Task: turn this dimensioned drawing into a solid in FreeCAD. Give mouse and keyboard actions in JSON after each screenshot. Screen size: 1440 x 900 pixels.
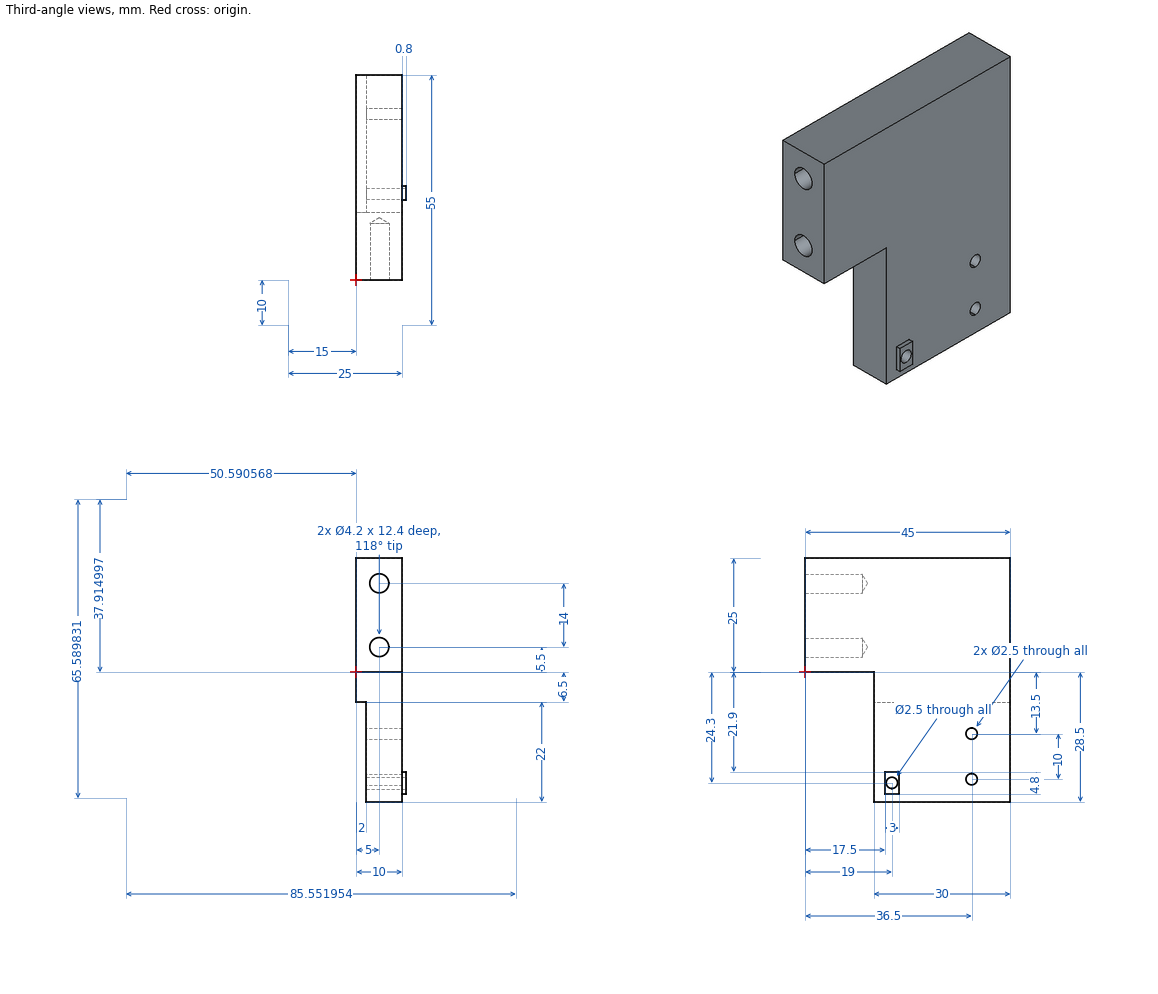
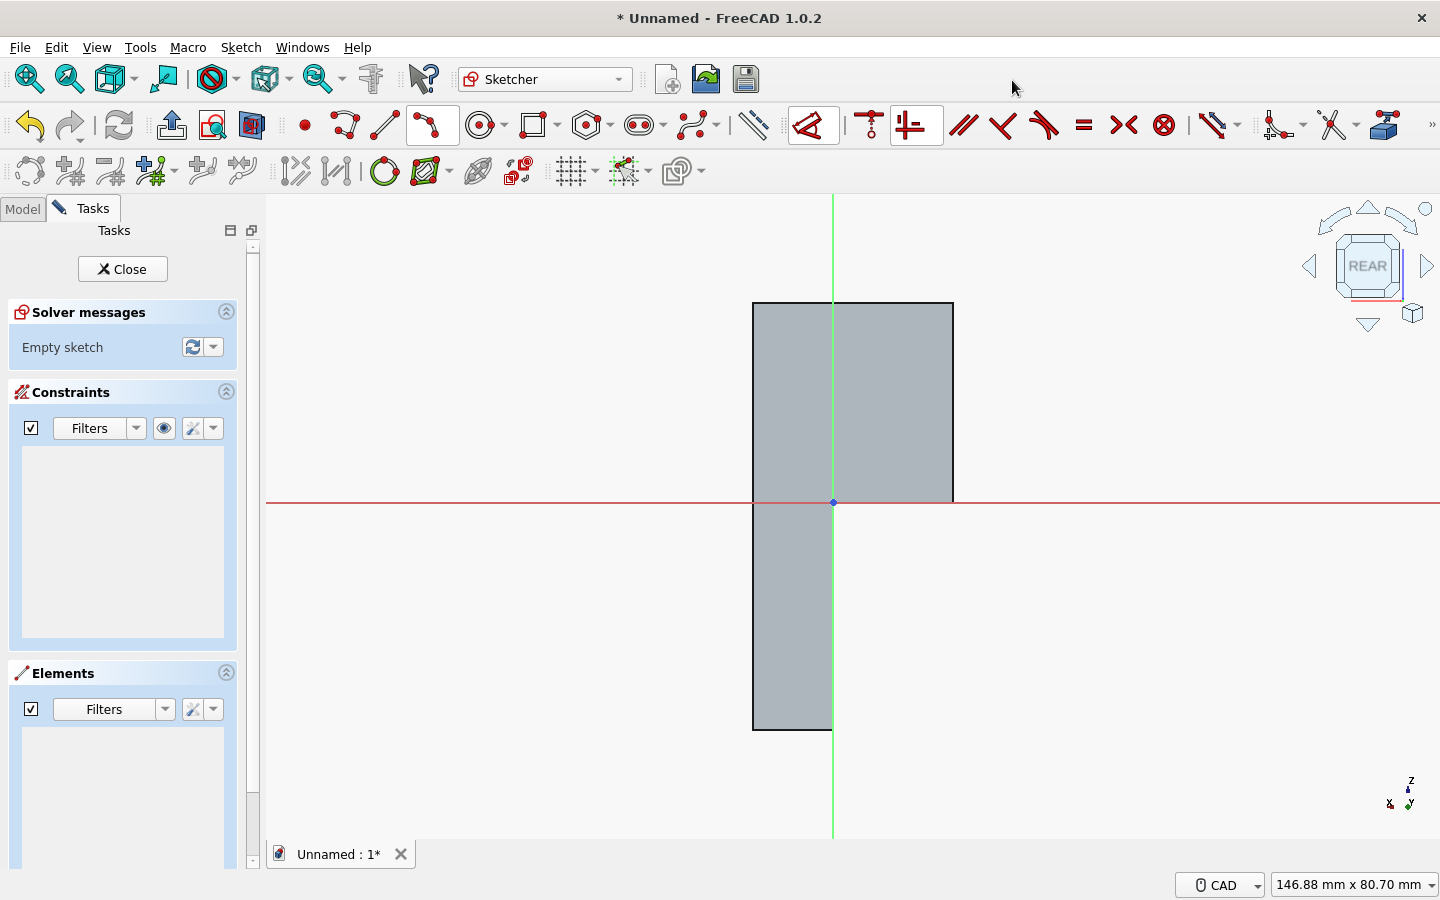
{"action": "scroll", "coordinate": [874, 738], "scroll_direction": "up", "scroll_amount": 3}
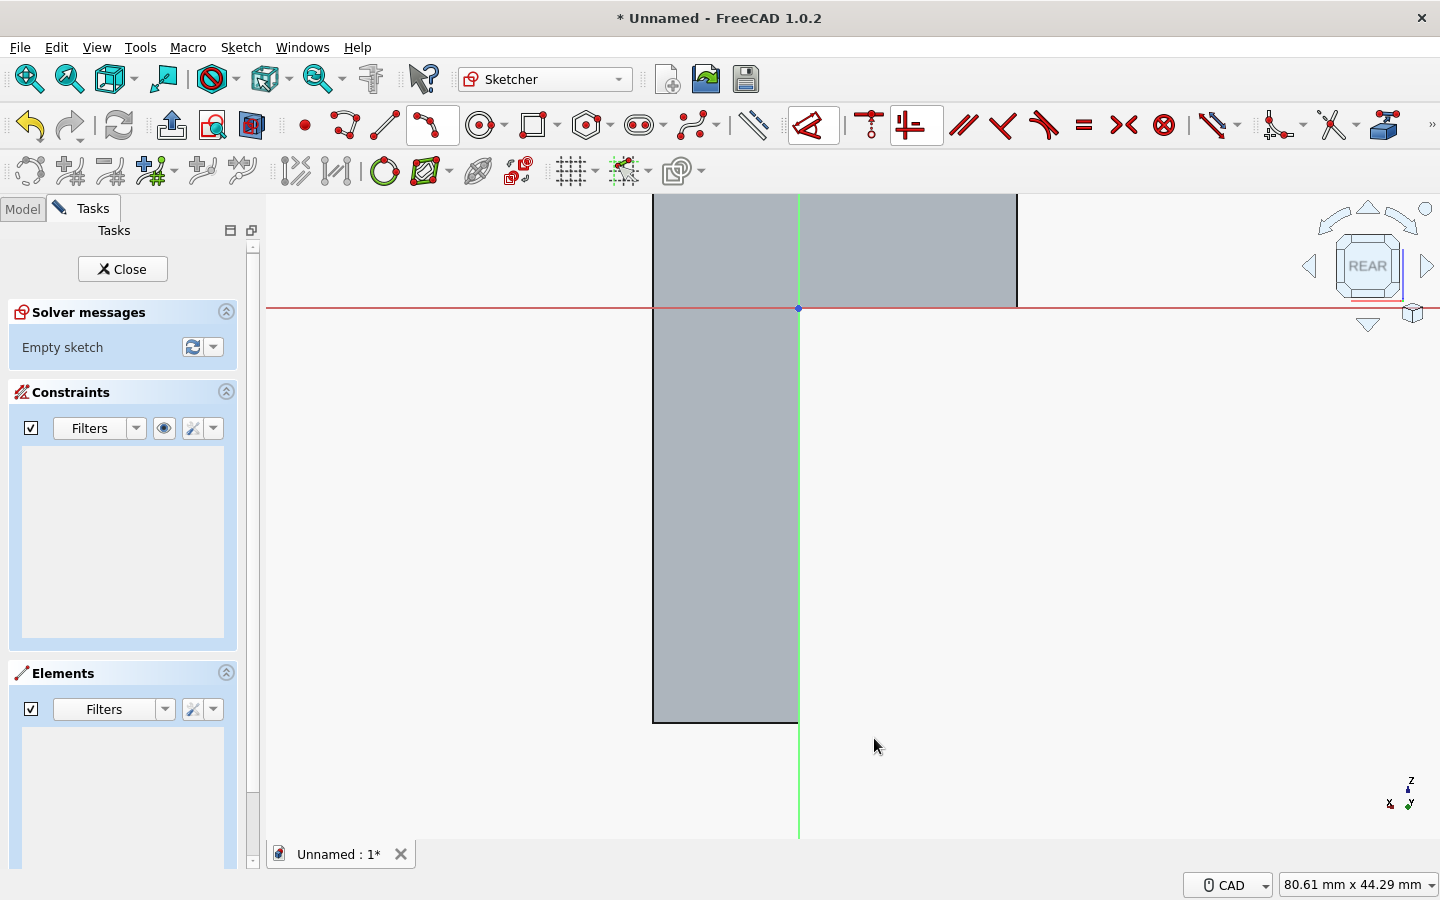
{"action": "key", "text": "g r"}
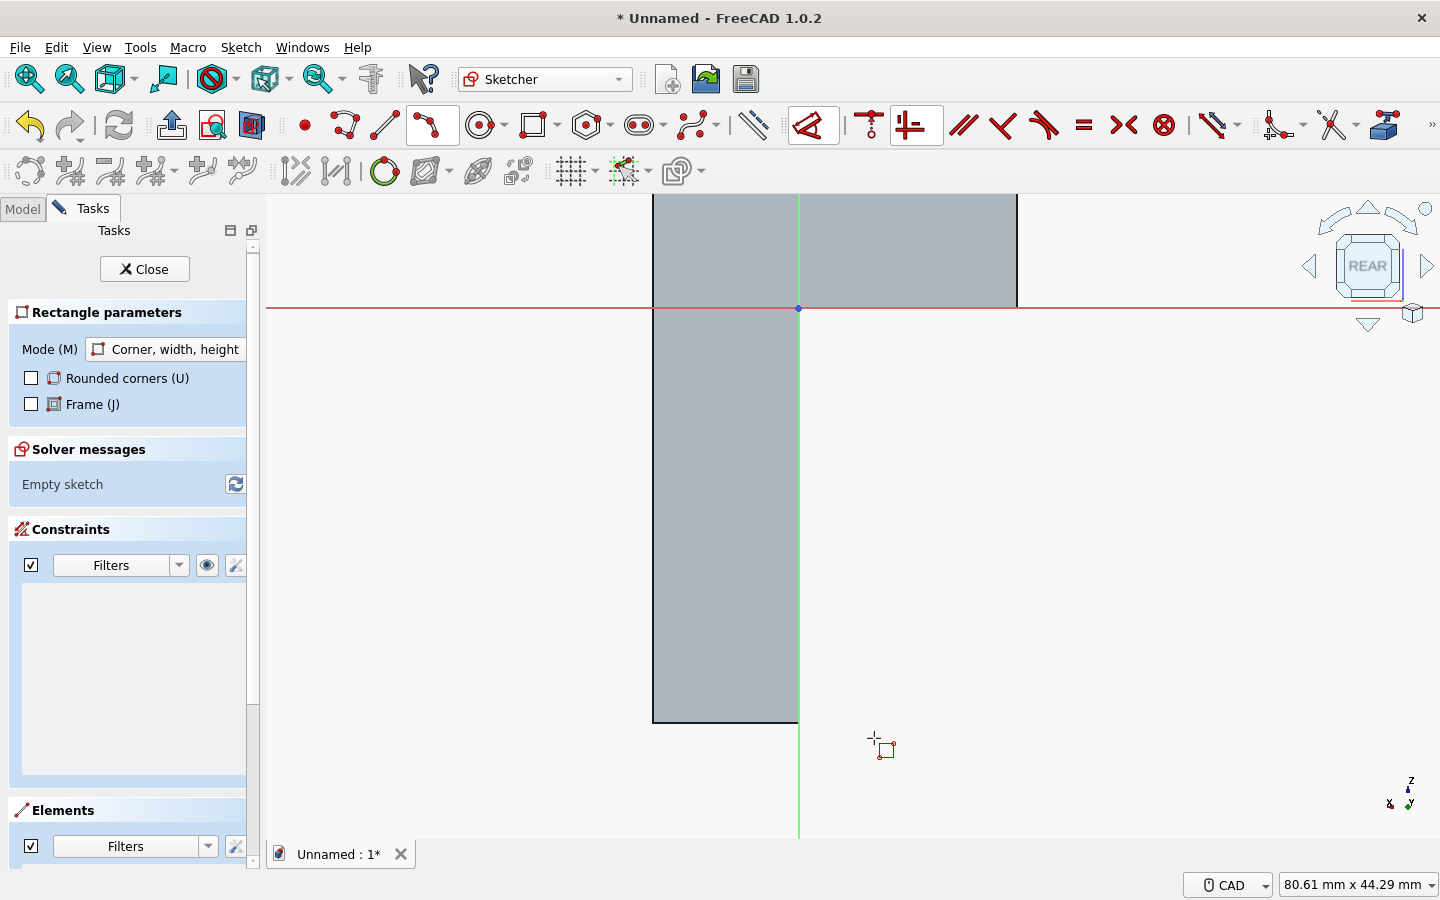
{"action": "left_click", "coordinate": [770, 403]}
{"action": "left_click", "coordinate": [799, 723]}
{"action": "key", "text": "Escape"}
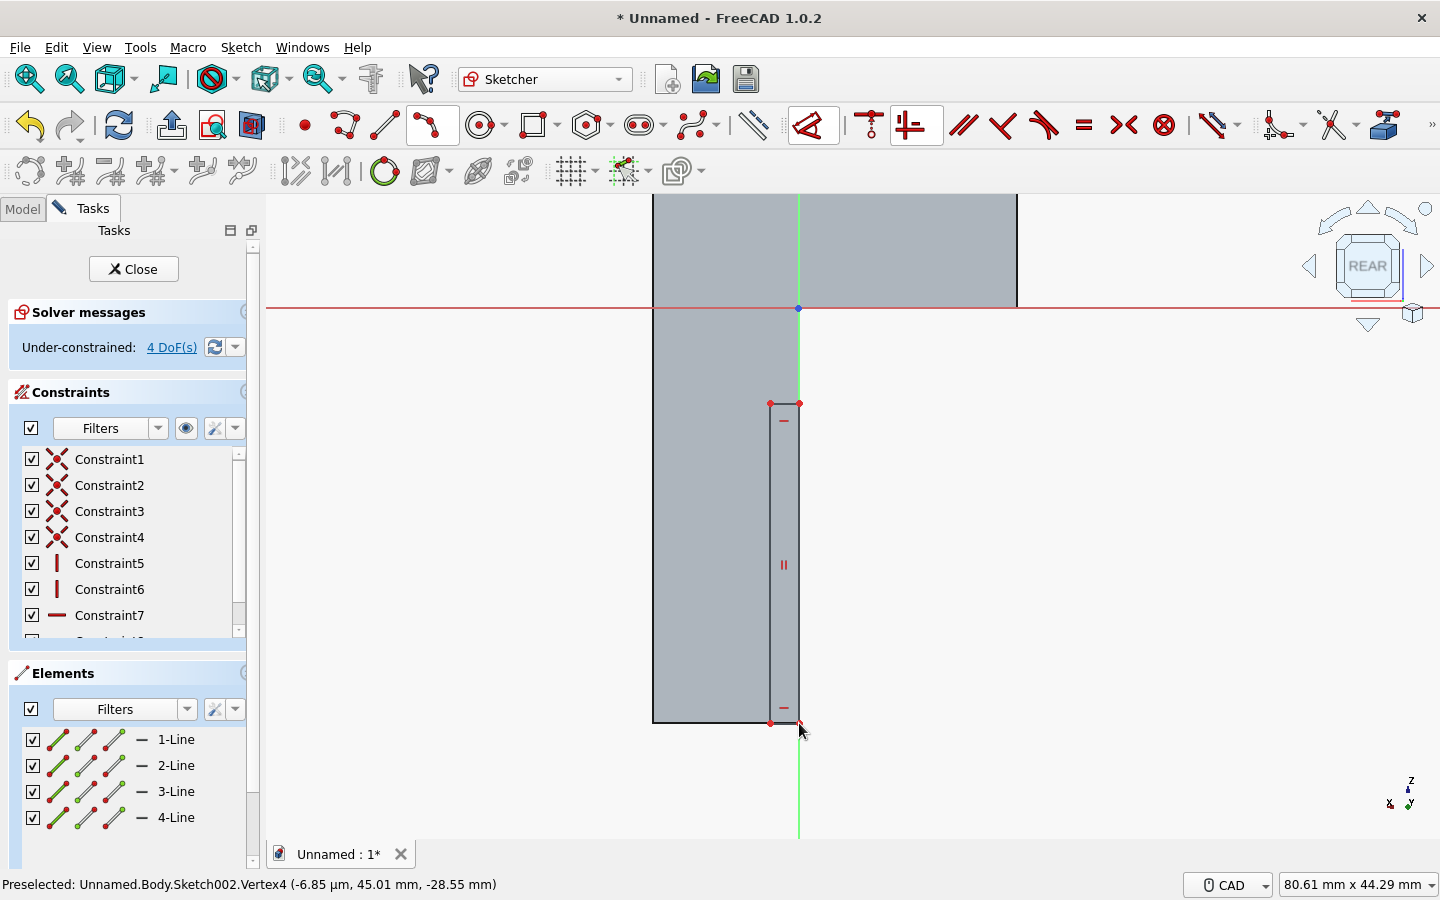
{"action": "left_click", "coordinate": [799, 724]}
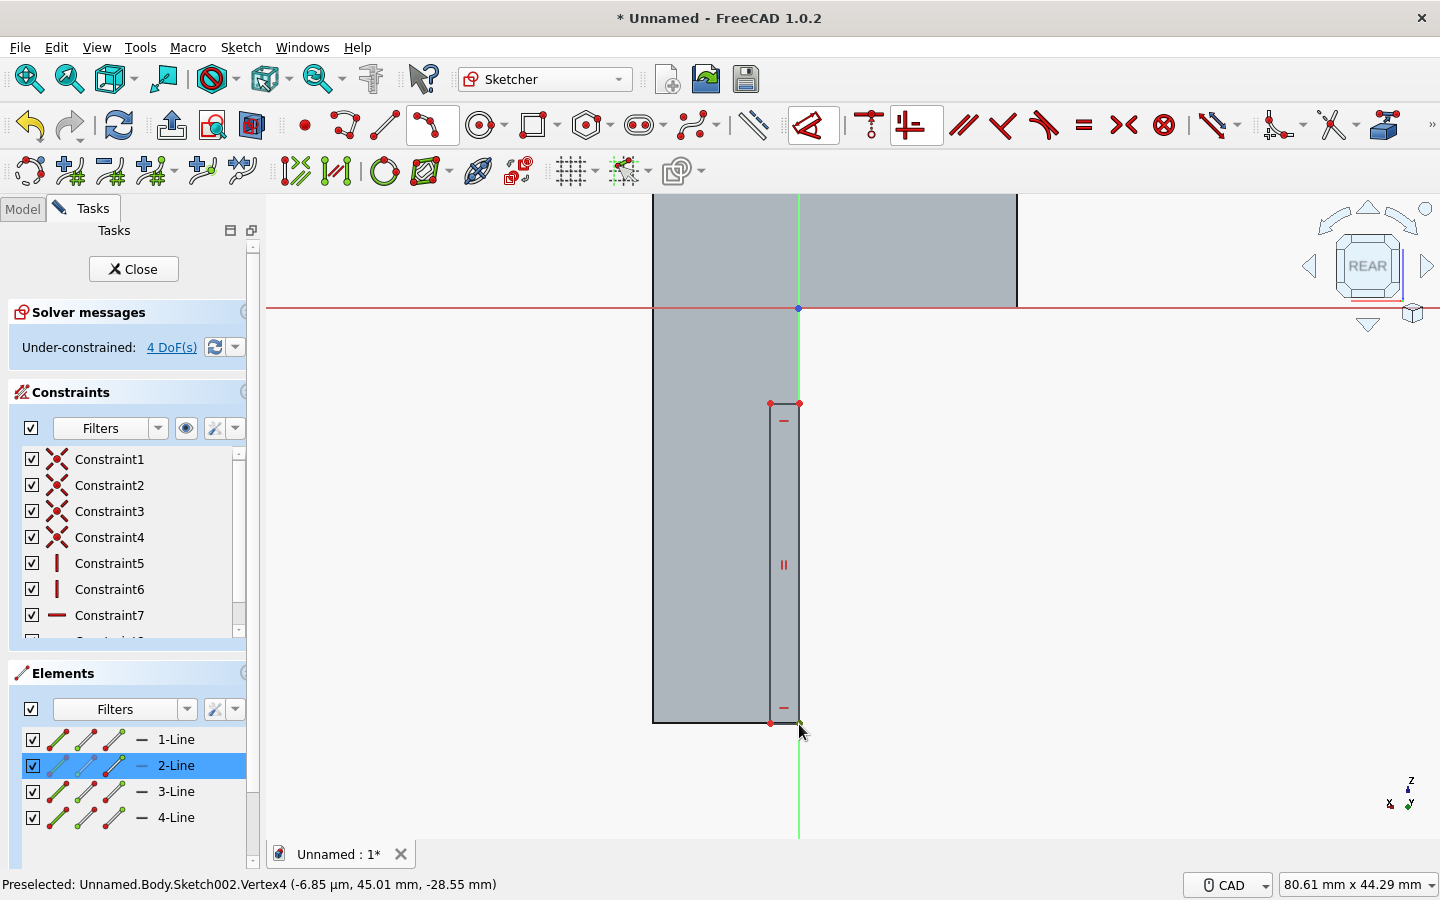
{"action": "left_click", "coordinate": [799, 769]}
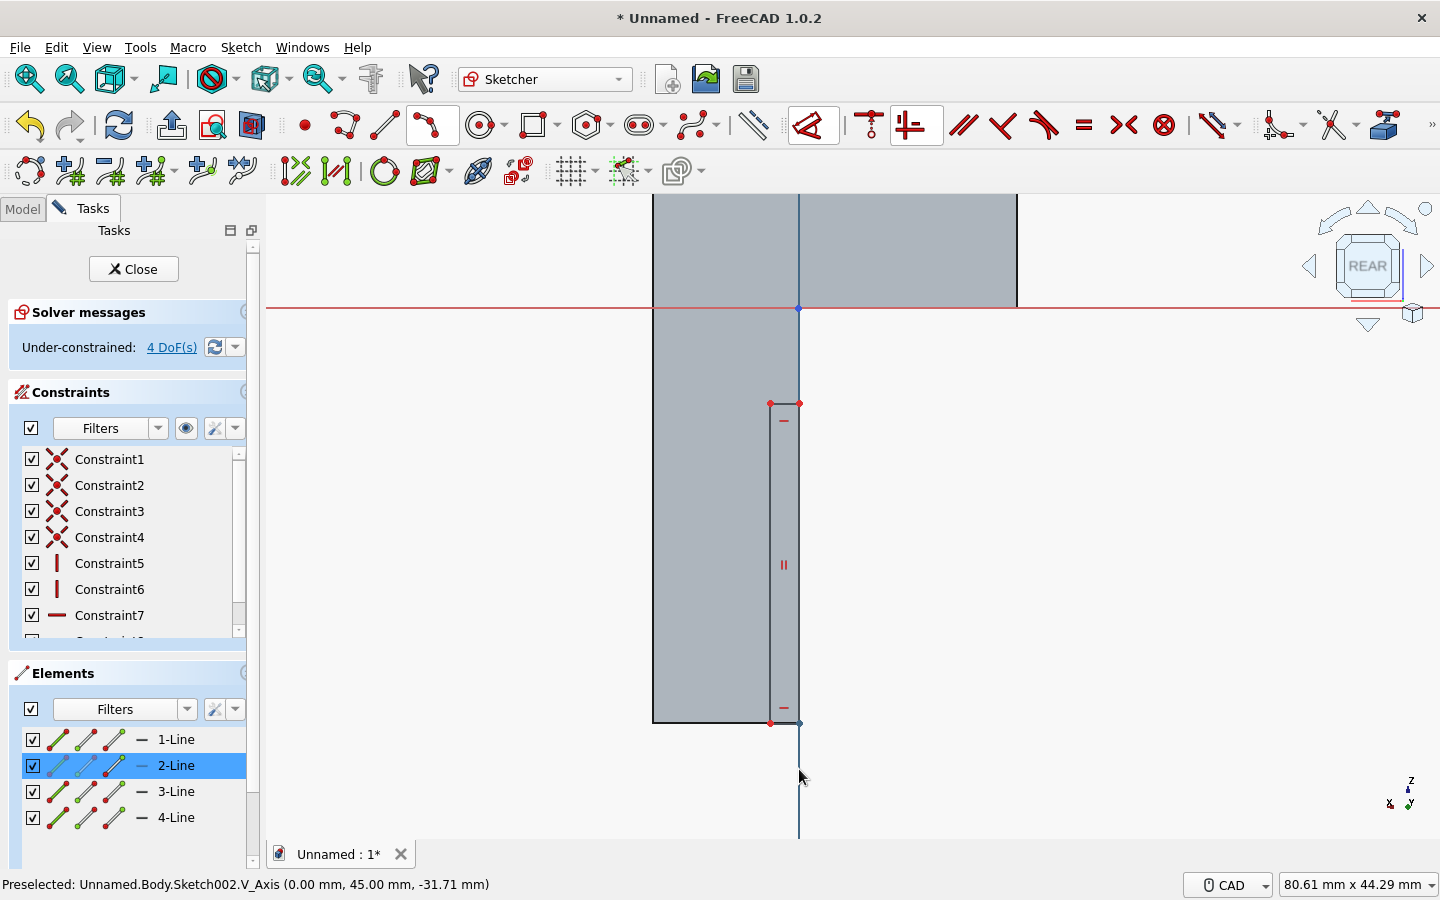
{"action": "left_click", "coordinate": [870, 126]}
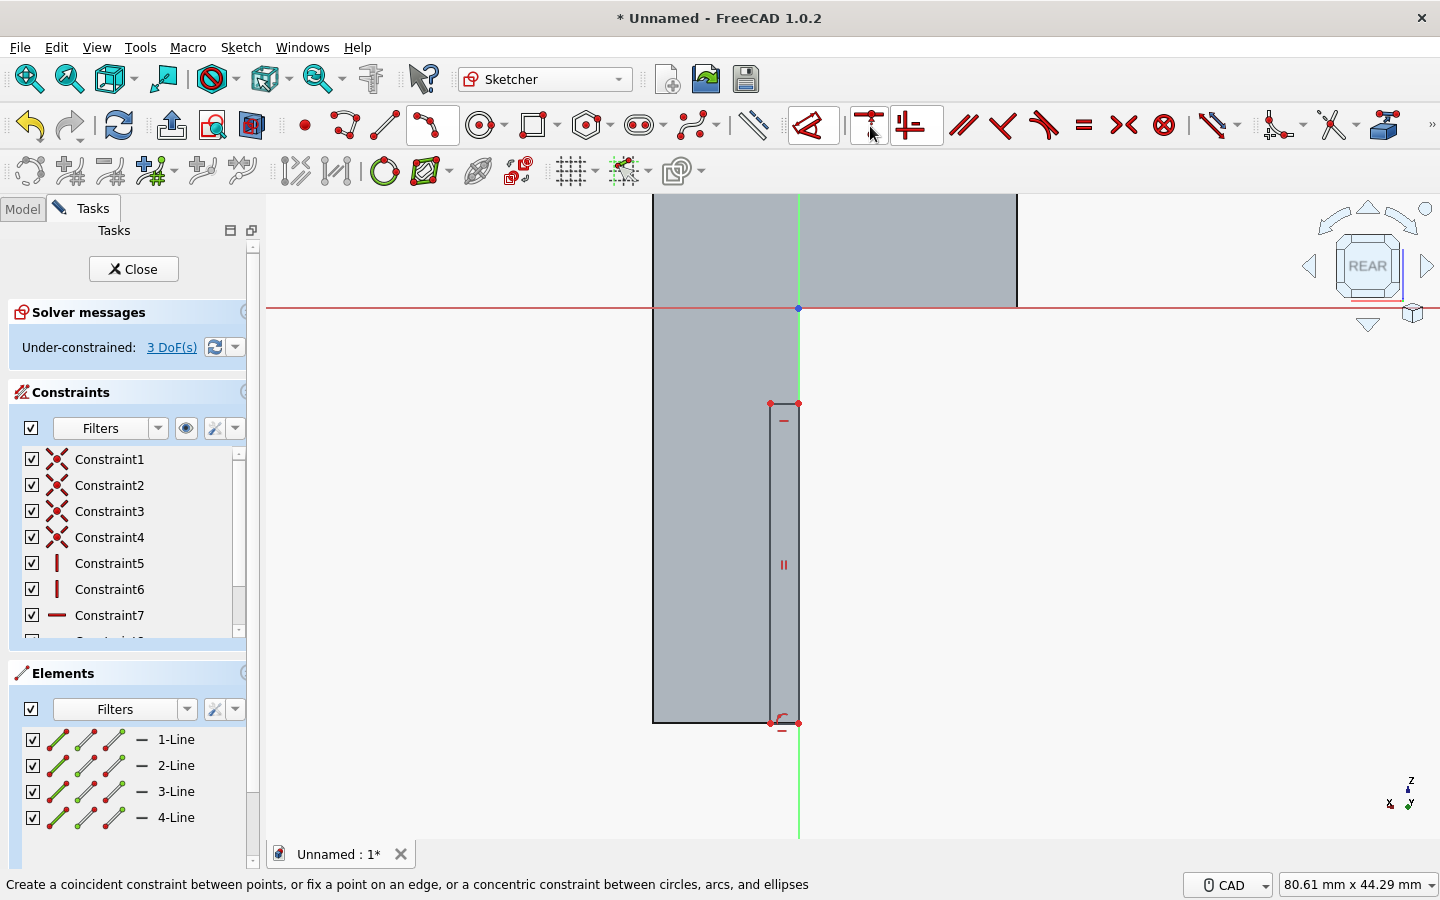
{"action": "scroll", "coordinate": [782, 724], "scroll_direction": "up", "scroll_amount": 2}